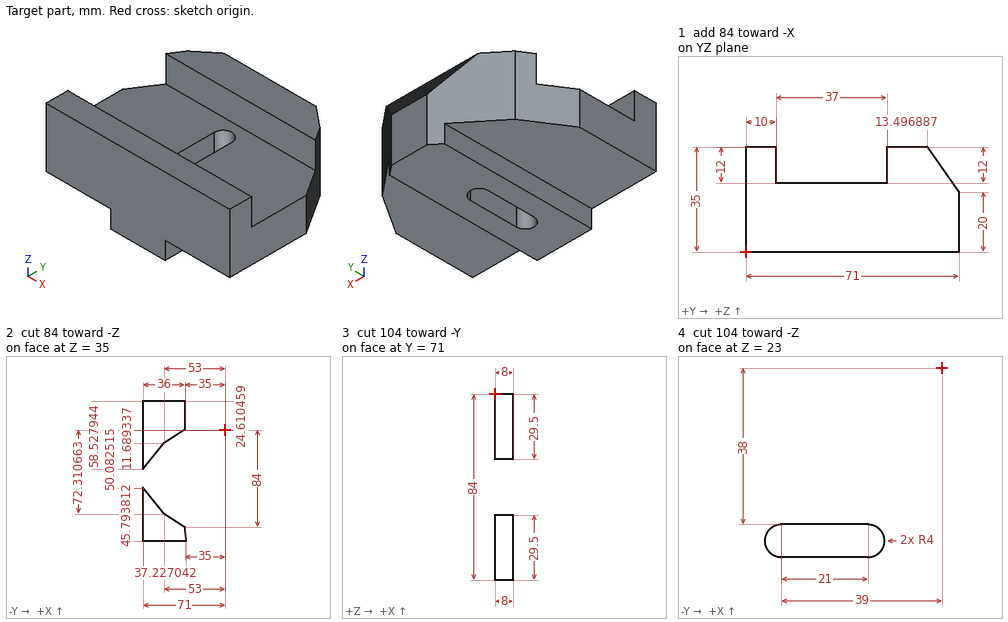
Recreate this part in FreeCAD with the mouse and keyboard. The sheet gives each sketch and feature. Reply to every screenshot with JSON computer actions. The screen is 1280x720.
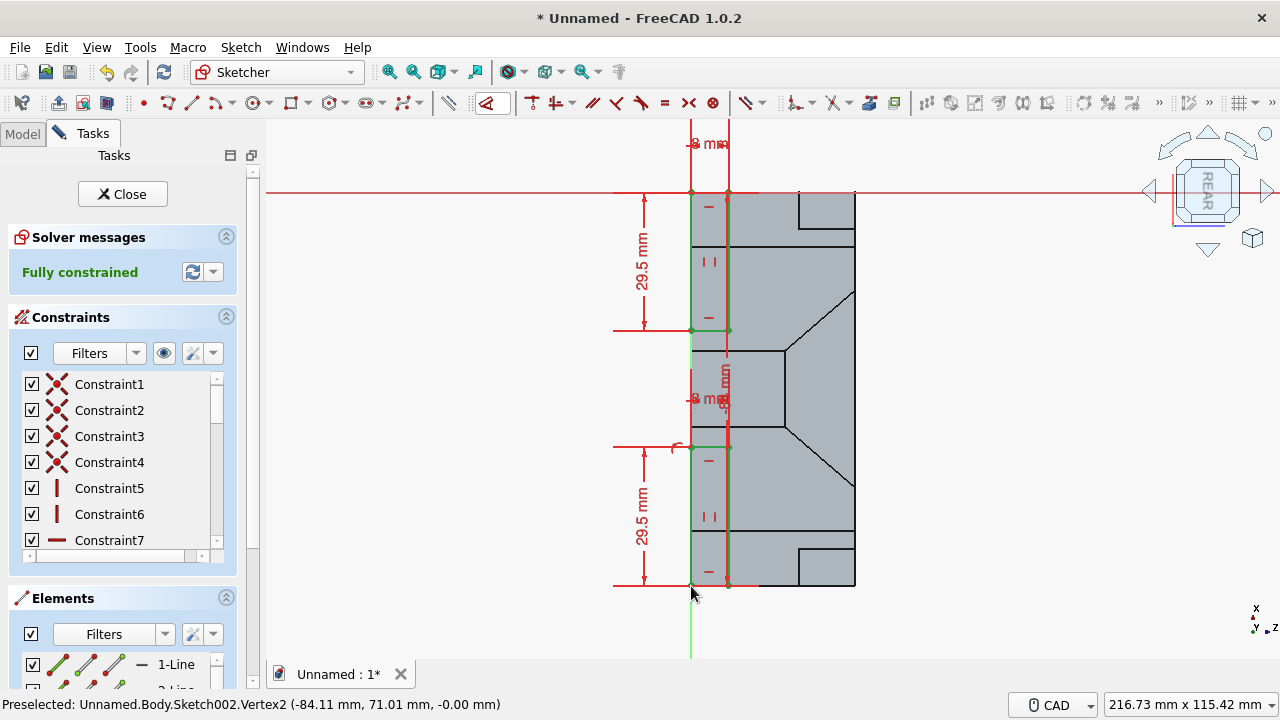
{"action": "left_click", "coordinate": [123, 194]}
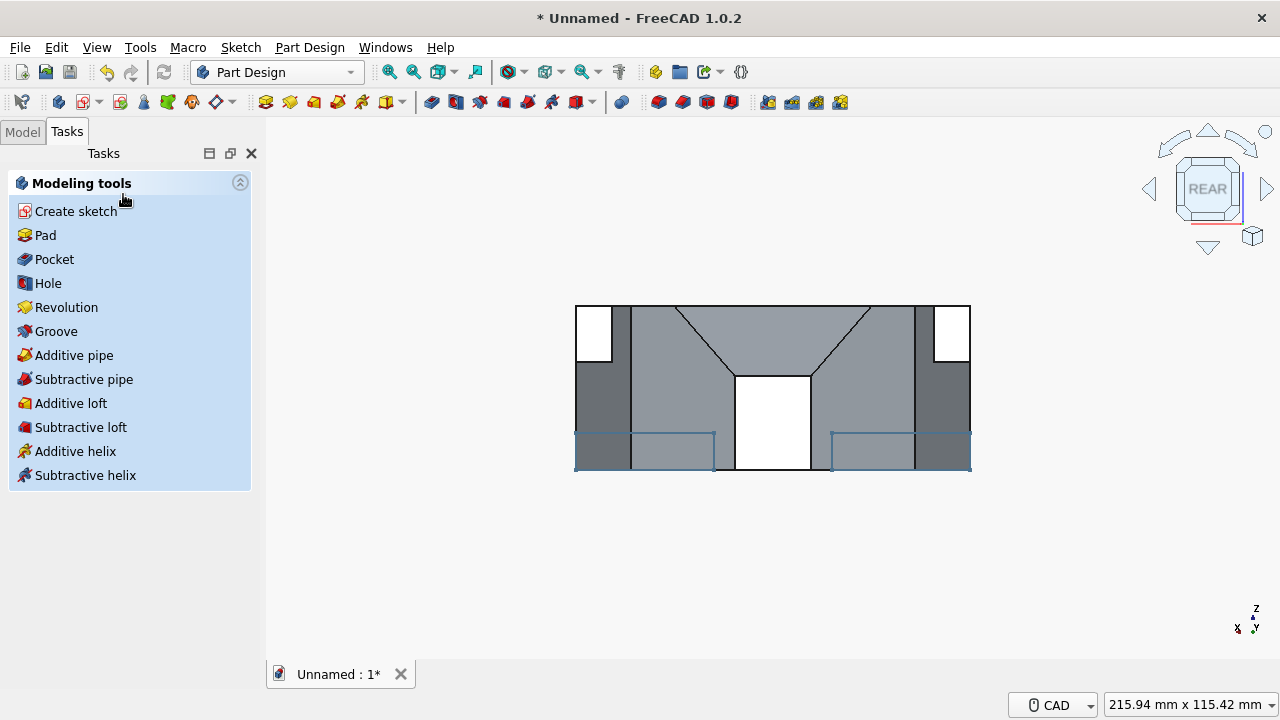
{"action": "left_click", "coordinate": [432, 102]}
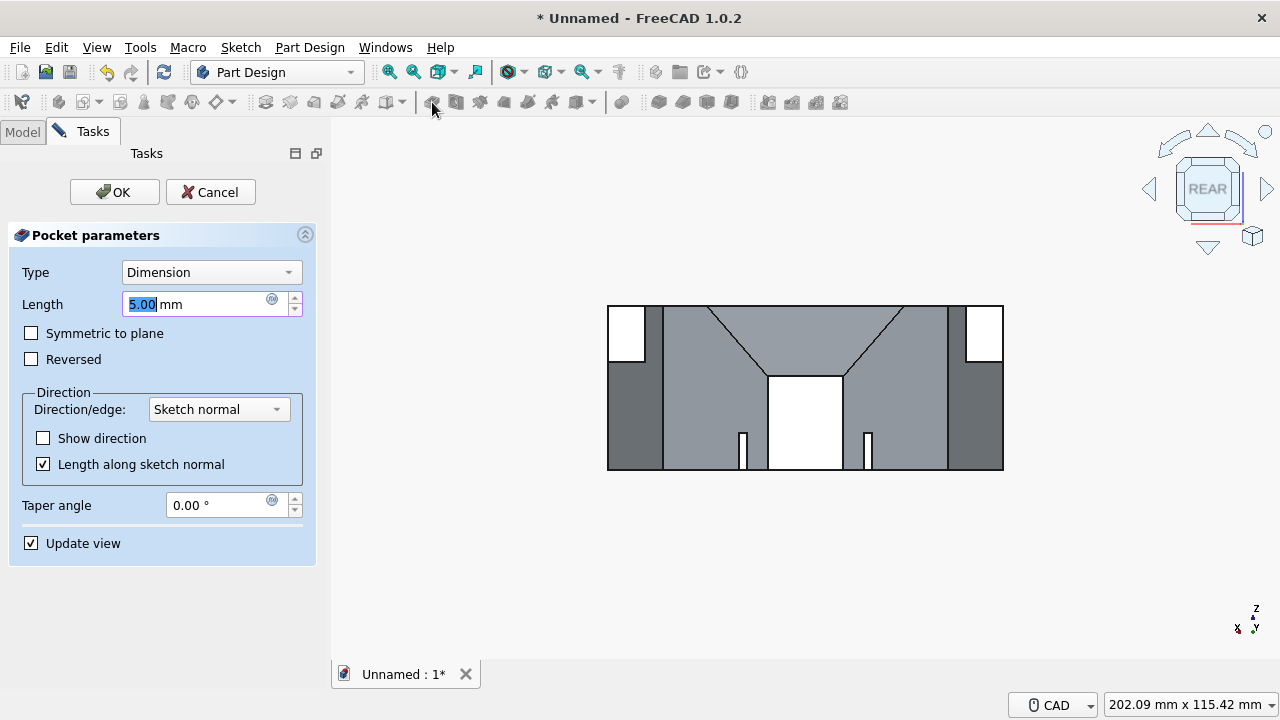
{"action": "type", "text": "104"}
{"action": "key", "text": "Tab"}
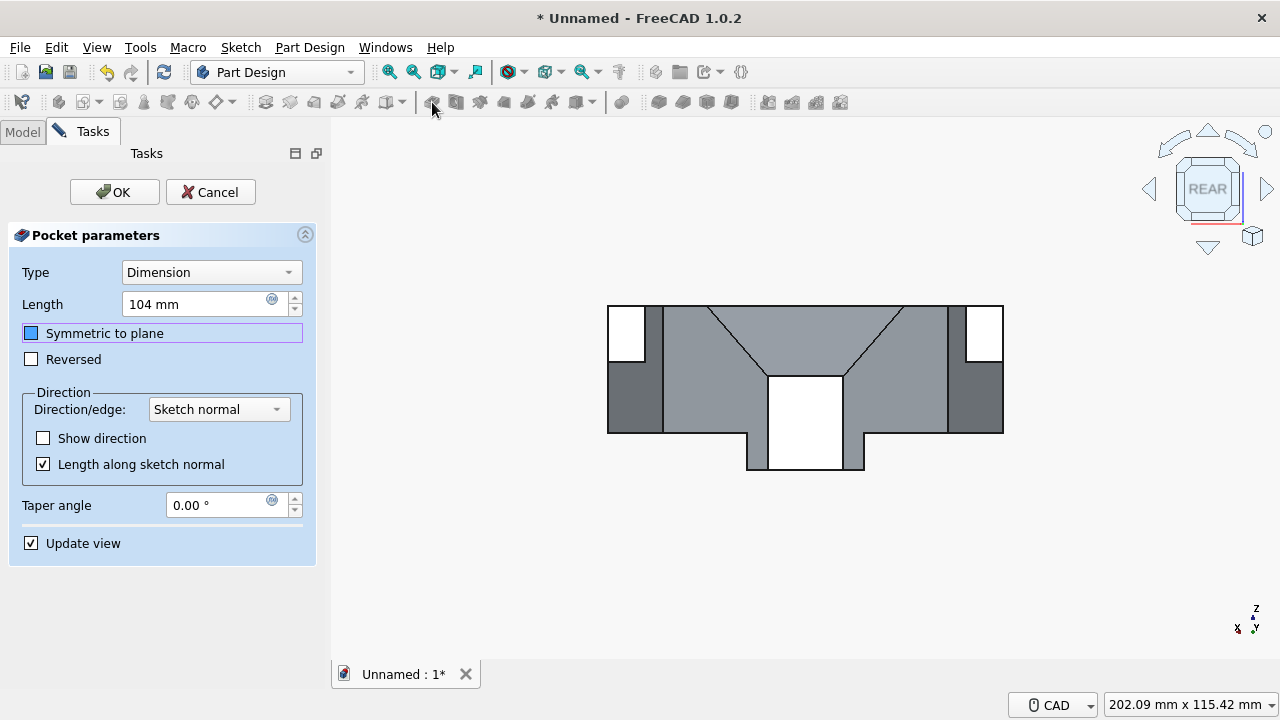
{"action": "left_click", "coordinate": [115, 192]}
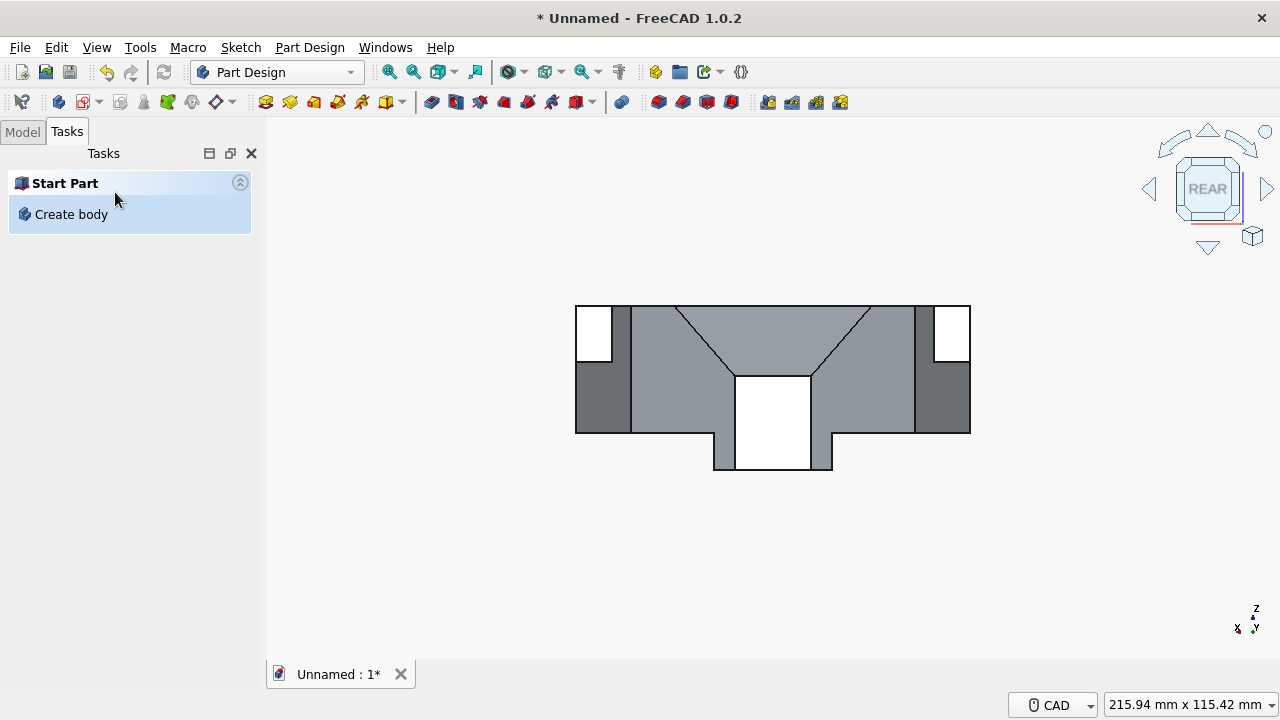
{"action": "left_click", "coordinate": [390, 72]}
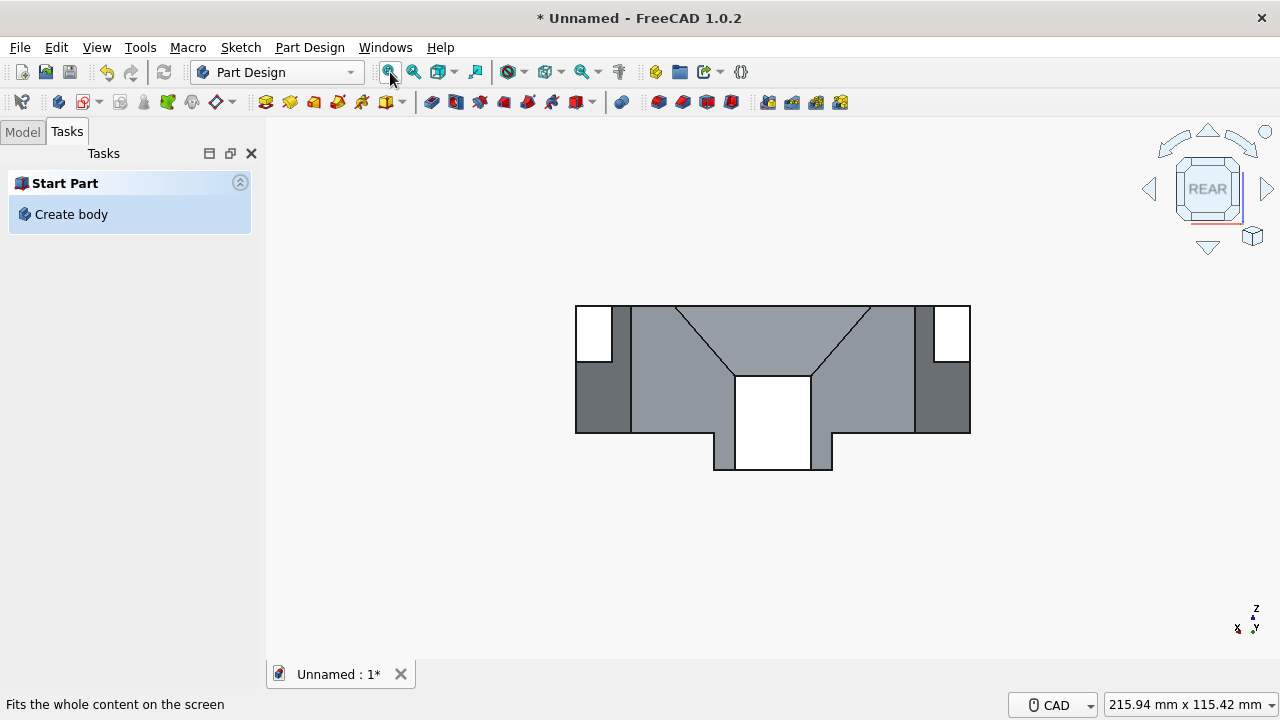
{"action": "key", "text": "0"}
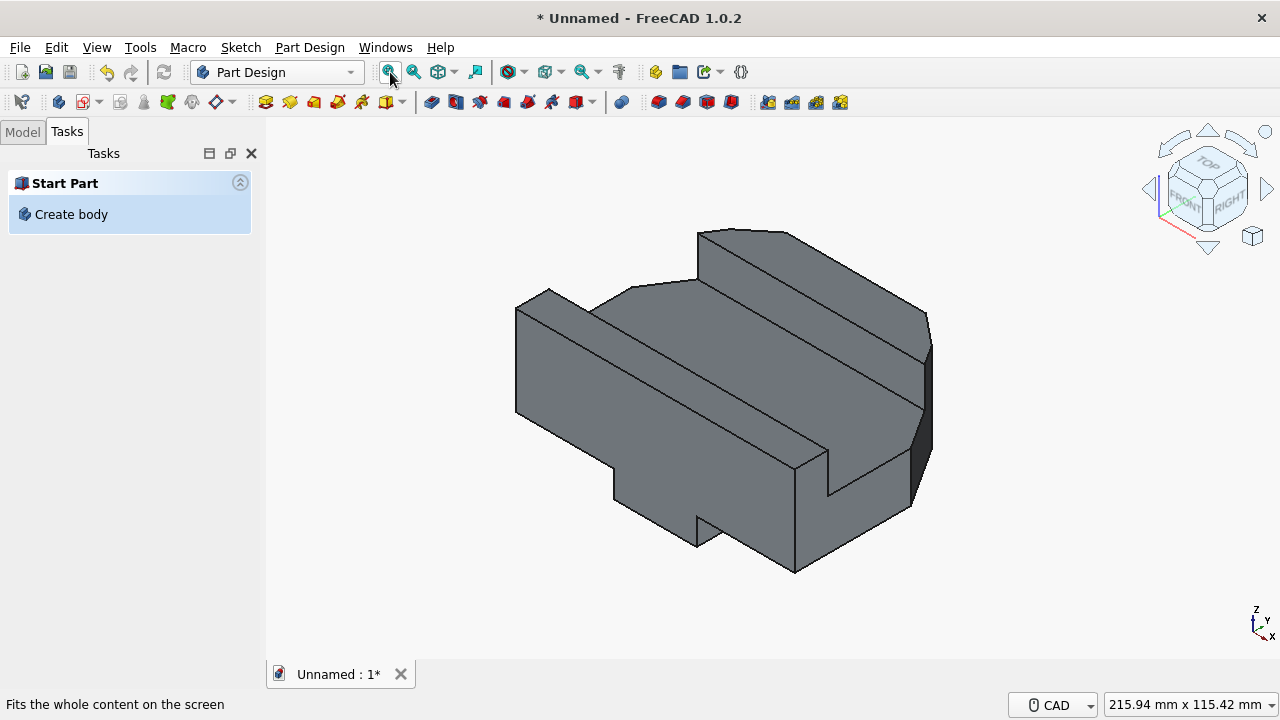
{"action": "left_click", "coordinate": [750, 379]}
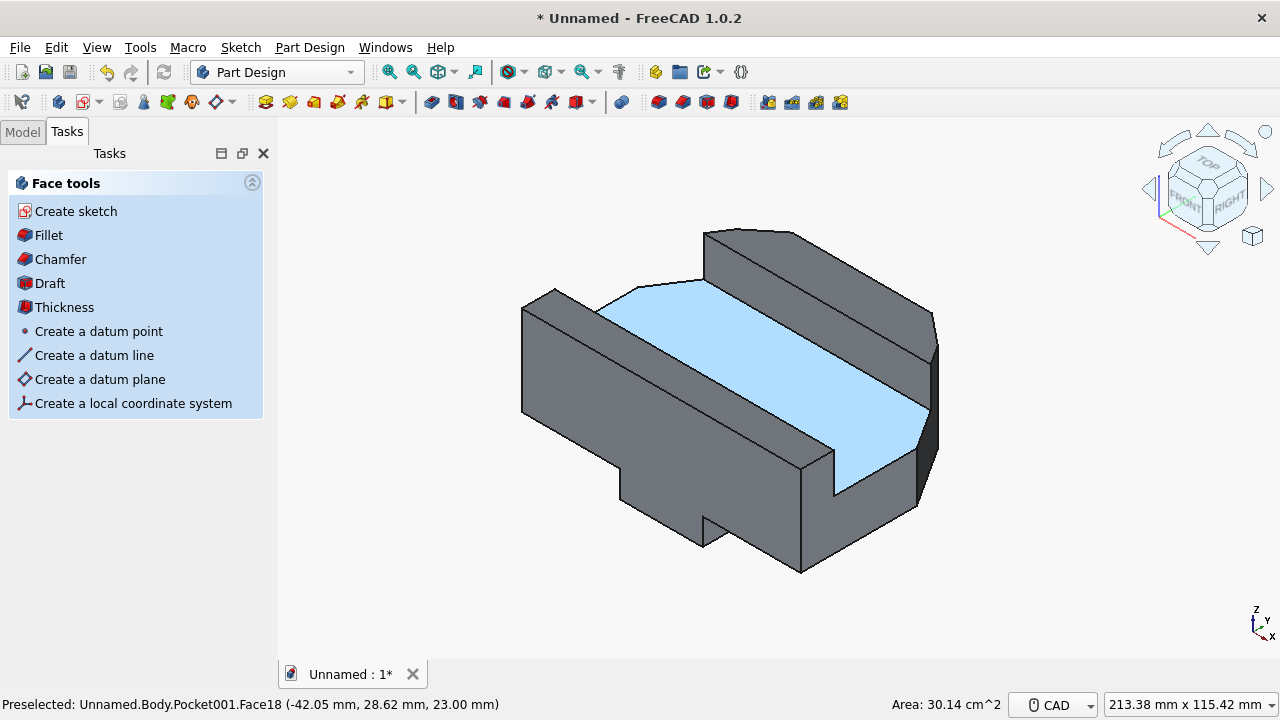
{"action": "left_click", "coordinate": [84, 102]}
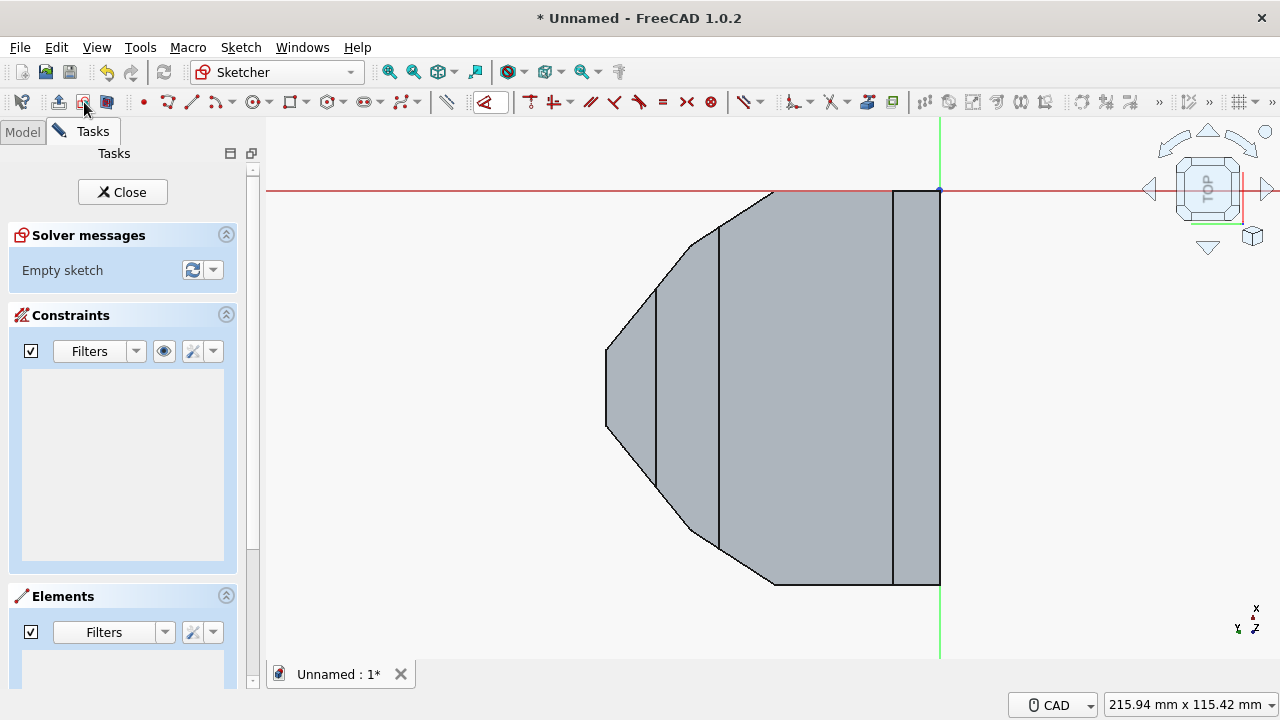
{"action": "scroll", "coordinate": [1112, 145], "scroll_direction": "up", "scroll_amount": 2}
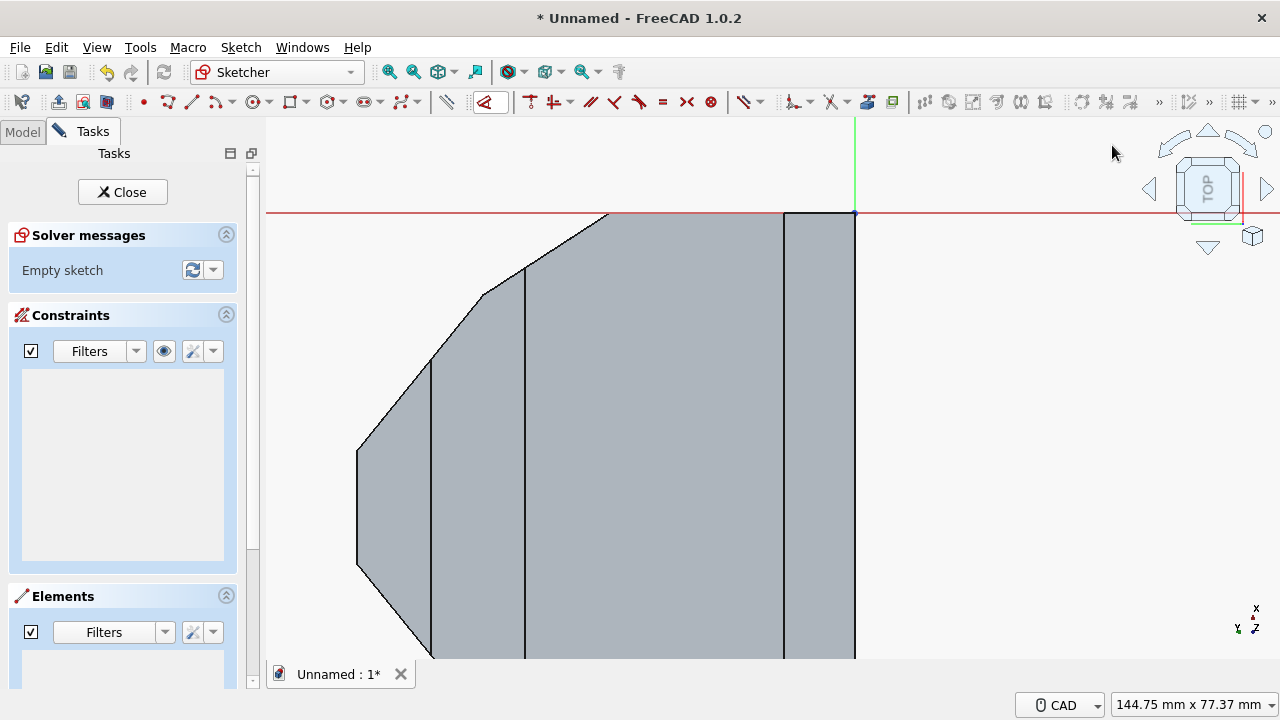
{"action": "left_click", "coordinate": [364, 102]}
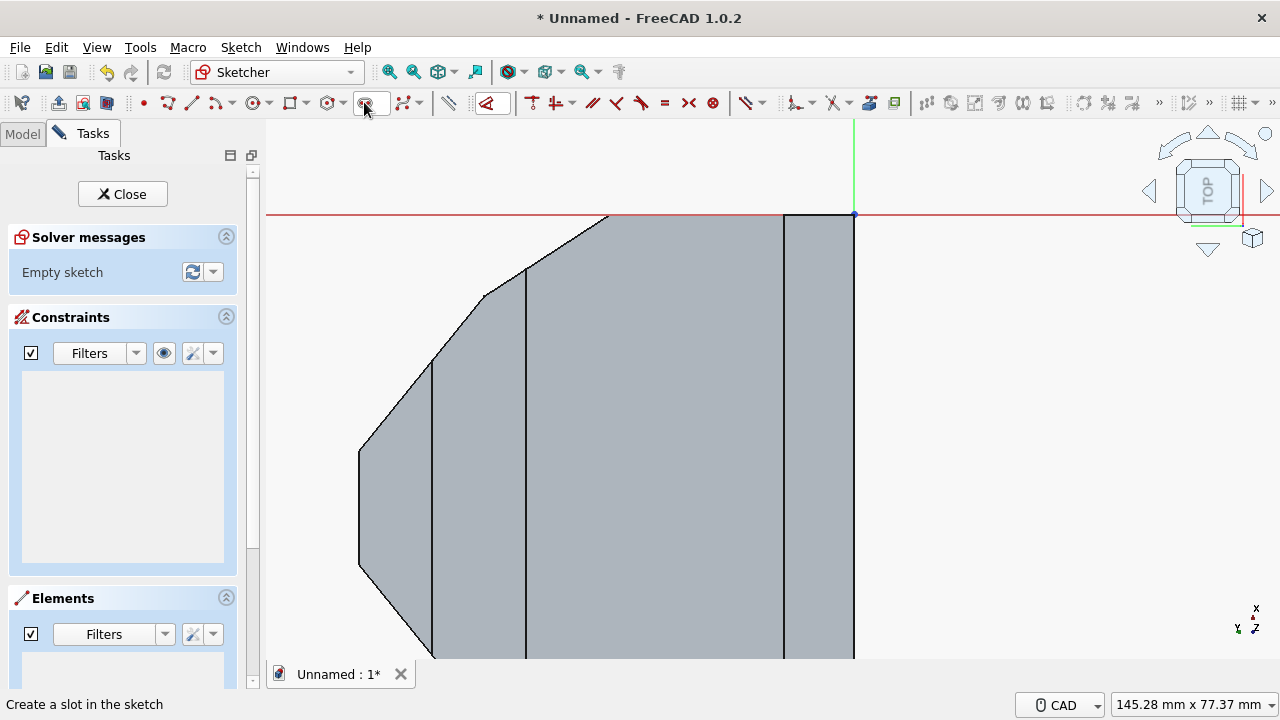
{"action": "left_click", "coordinate": [582, 508]}